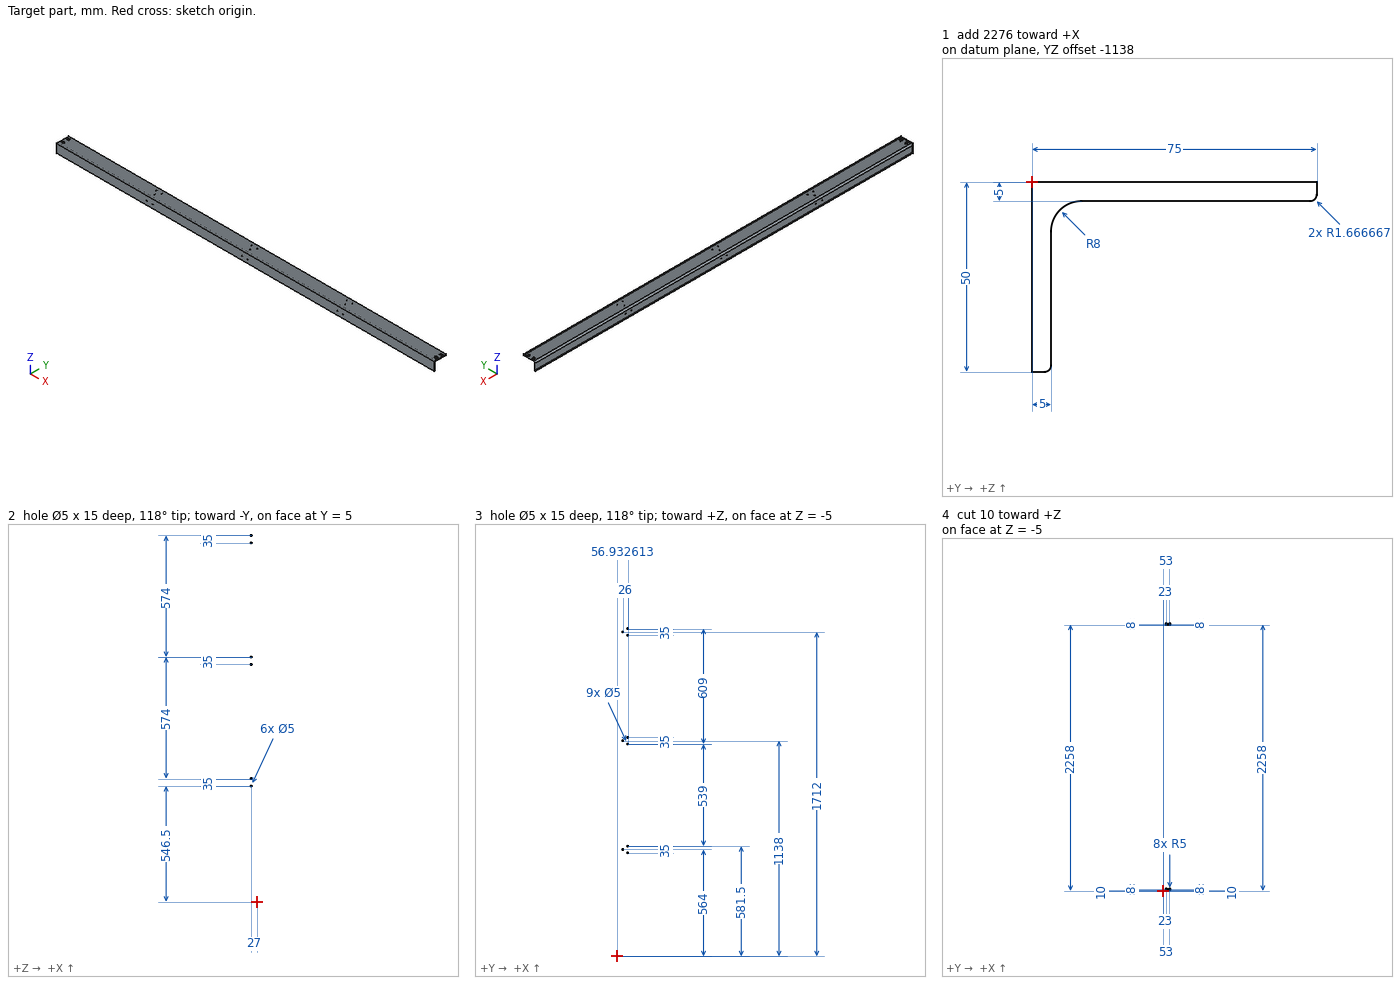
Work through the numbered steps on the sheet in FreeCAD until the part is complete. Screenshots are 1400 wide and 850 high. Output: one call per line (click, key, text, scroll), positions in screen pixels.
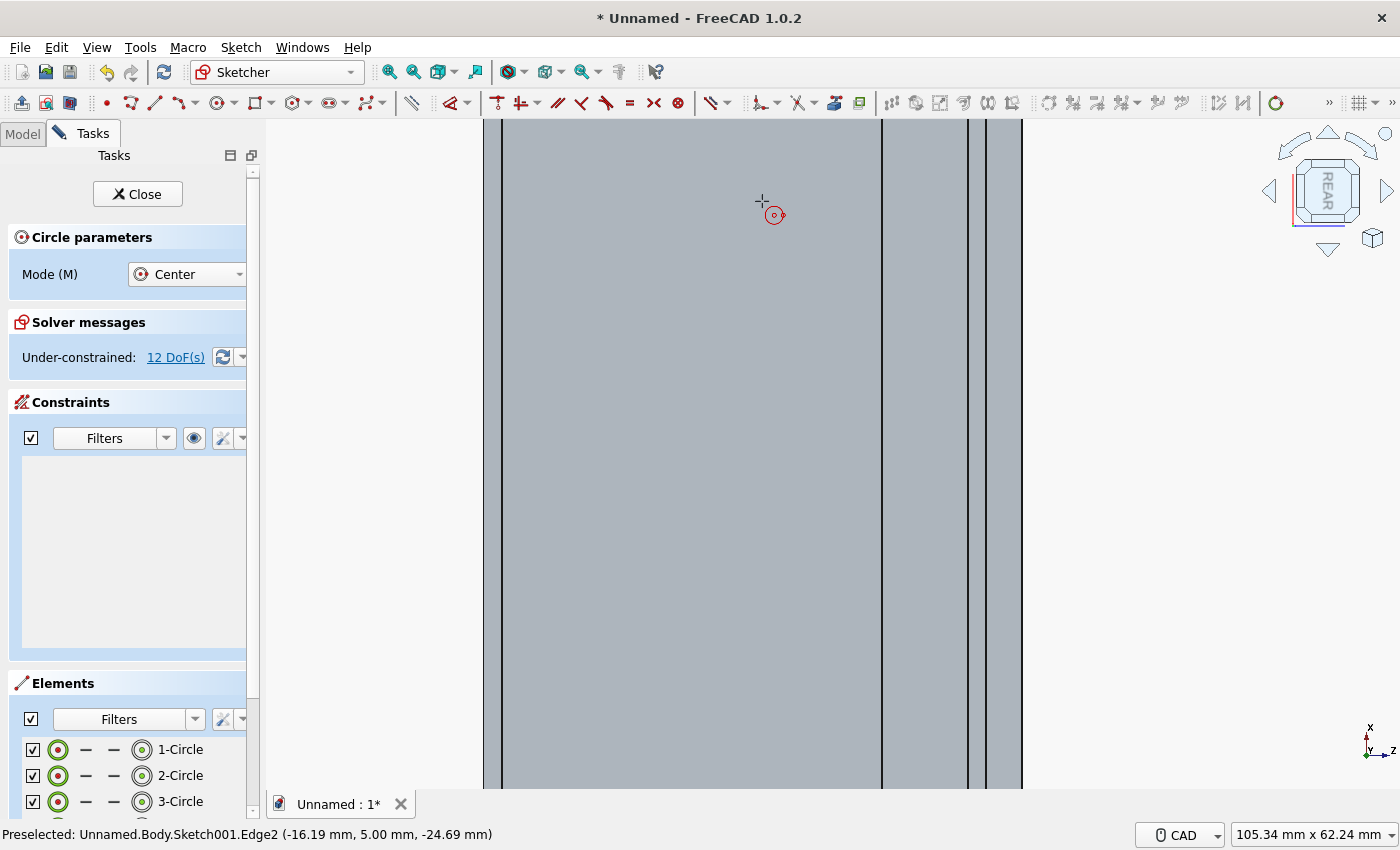
scroll(762, 200, down, 18)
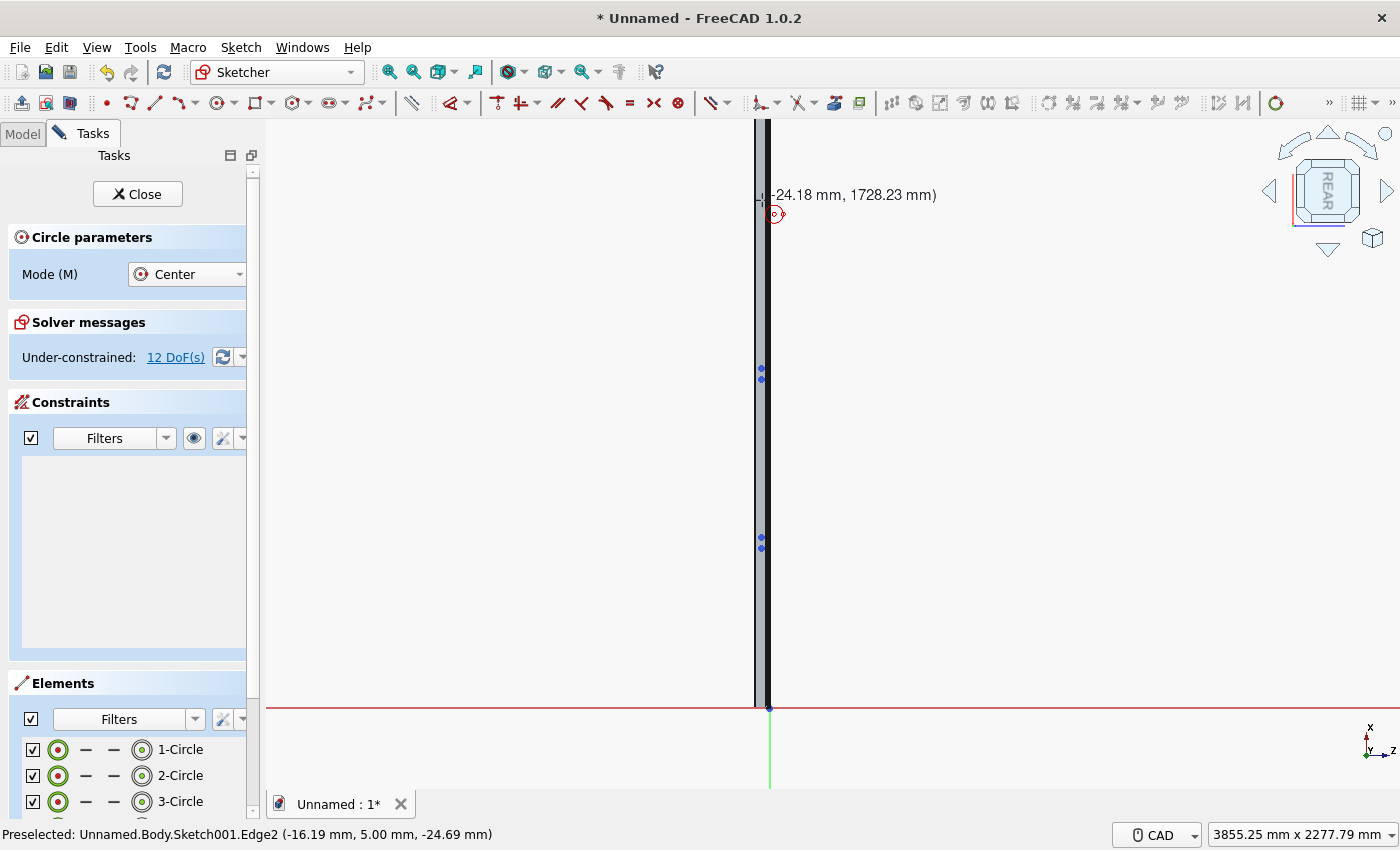
scroll(762, 200, up, 4)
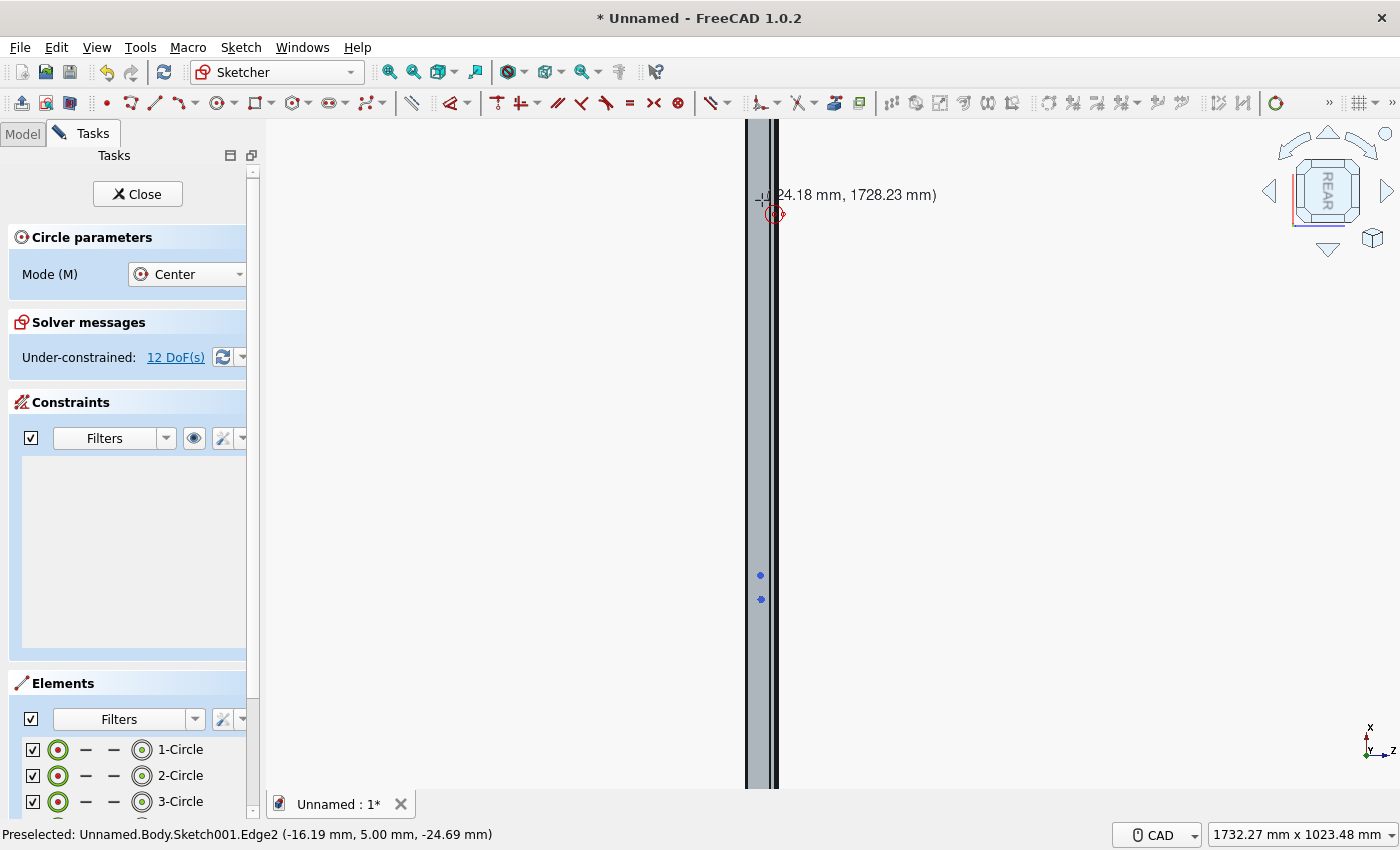
click(761, 199)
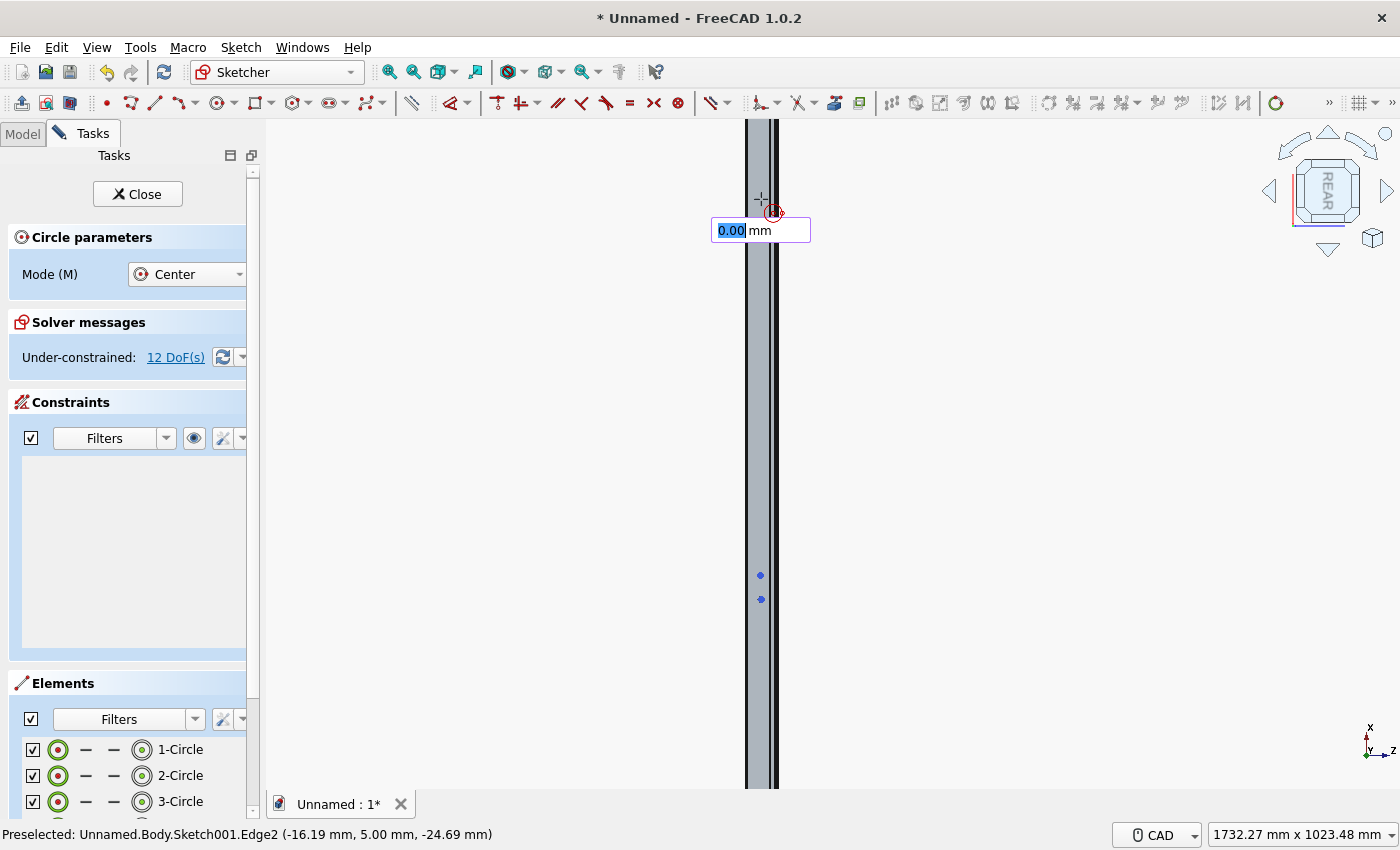
scroll(762, 198, up, 12)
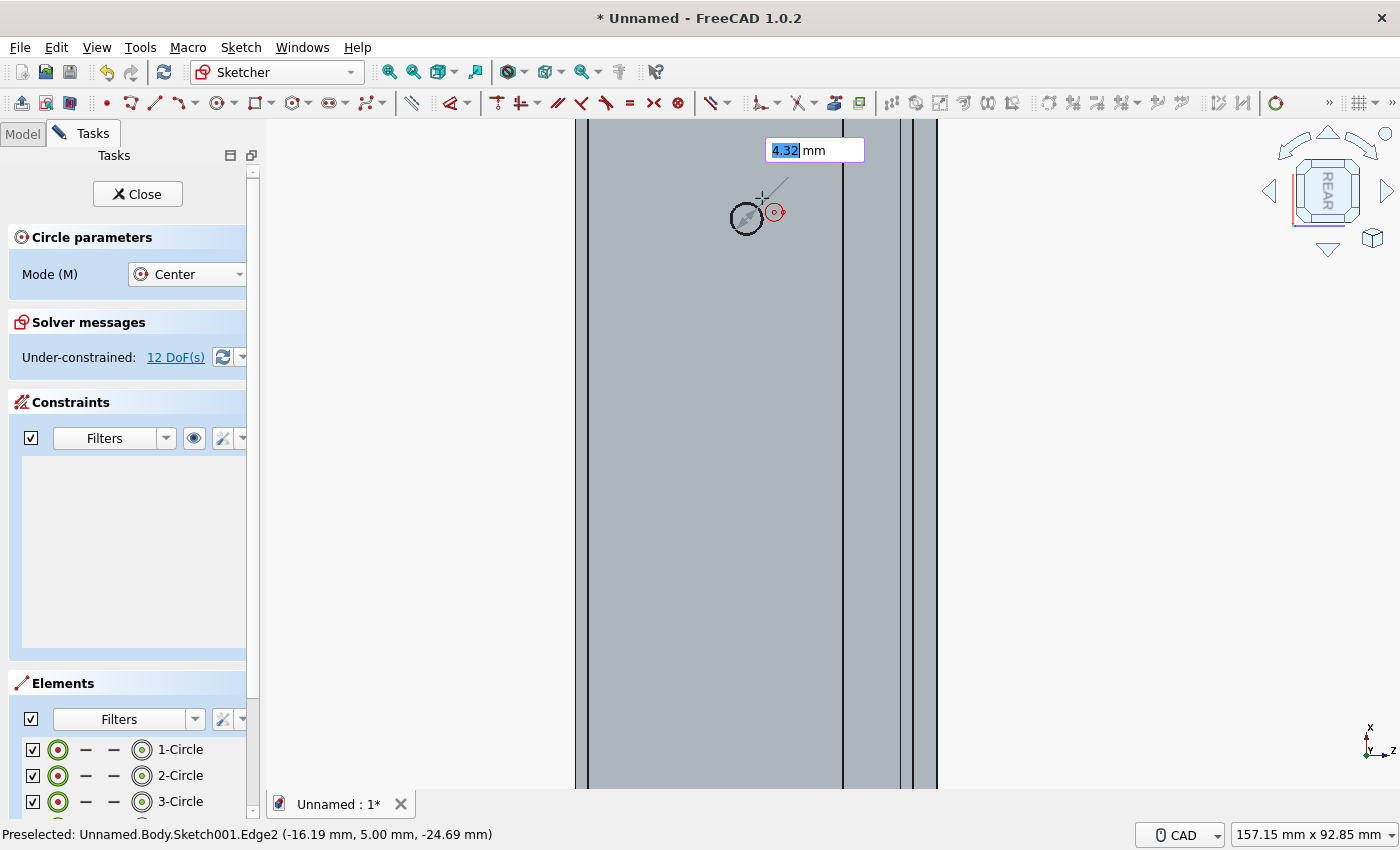
click(755, 199)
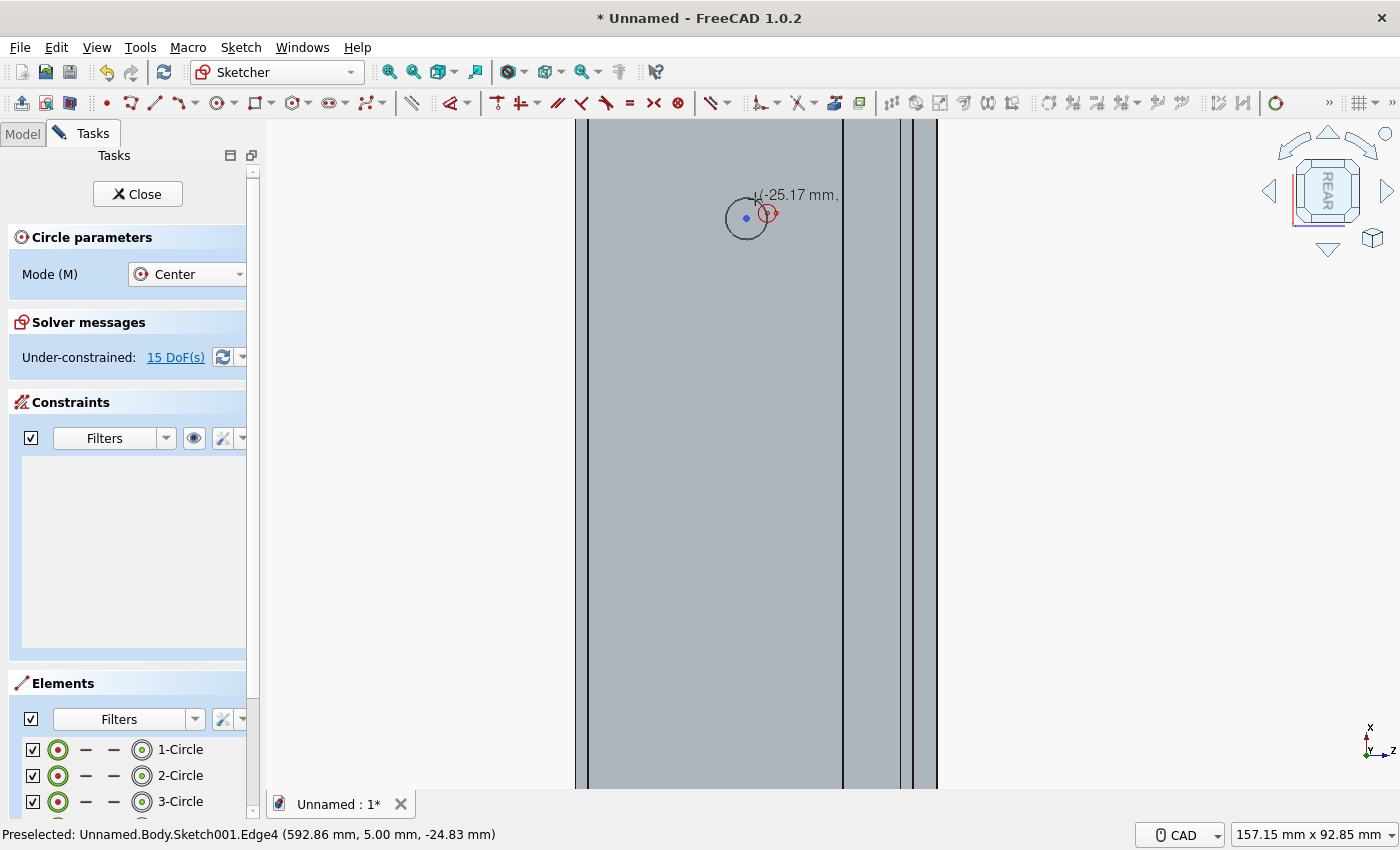
scroll(742, 464, up, 2)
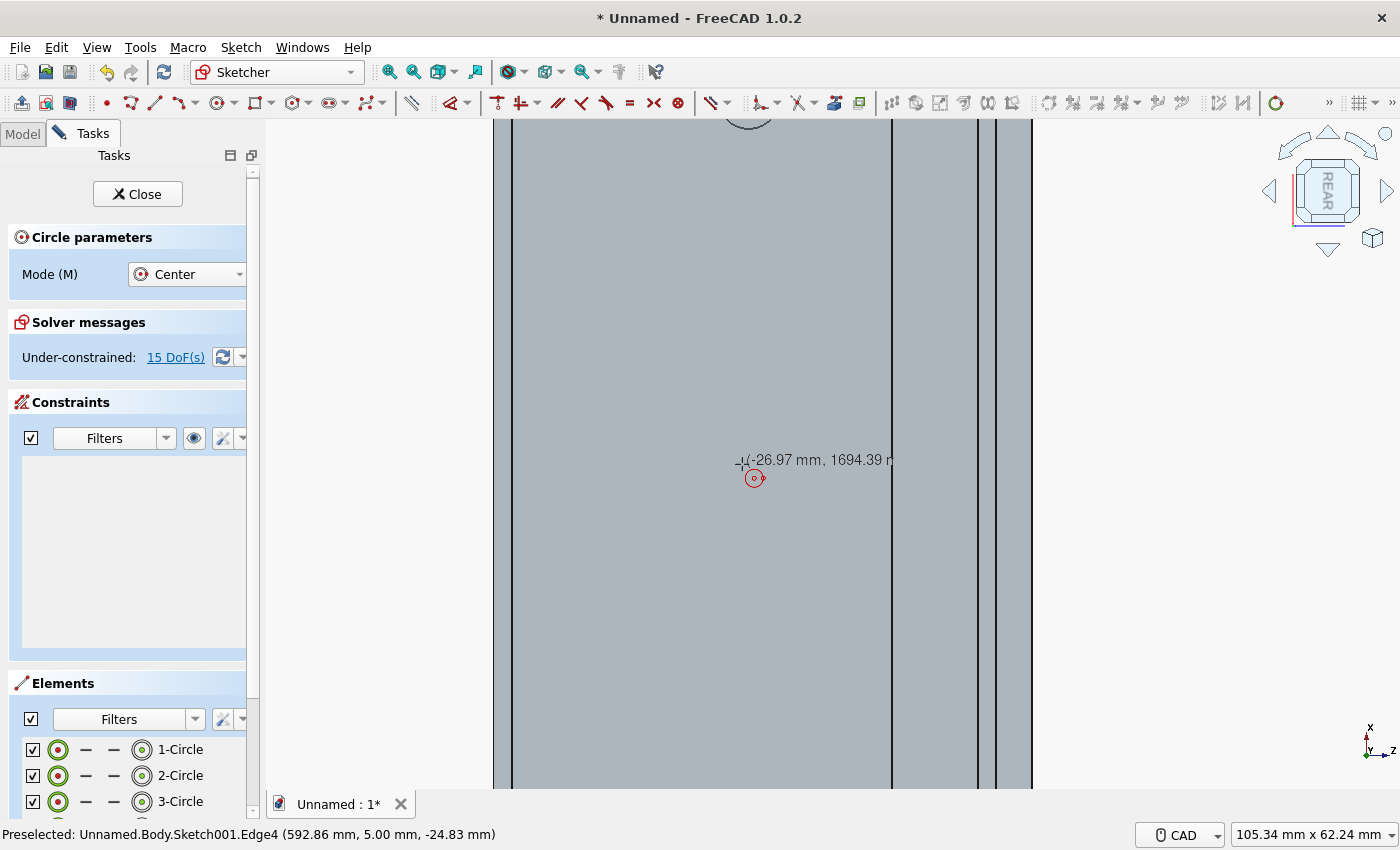
scroll(761, 203, down, 18)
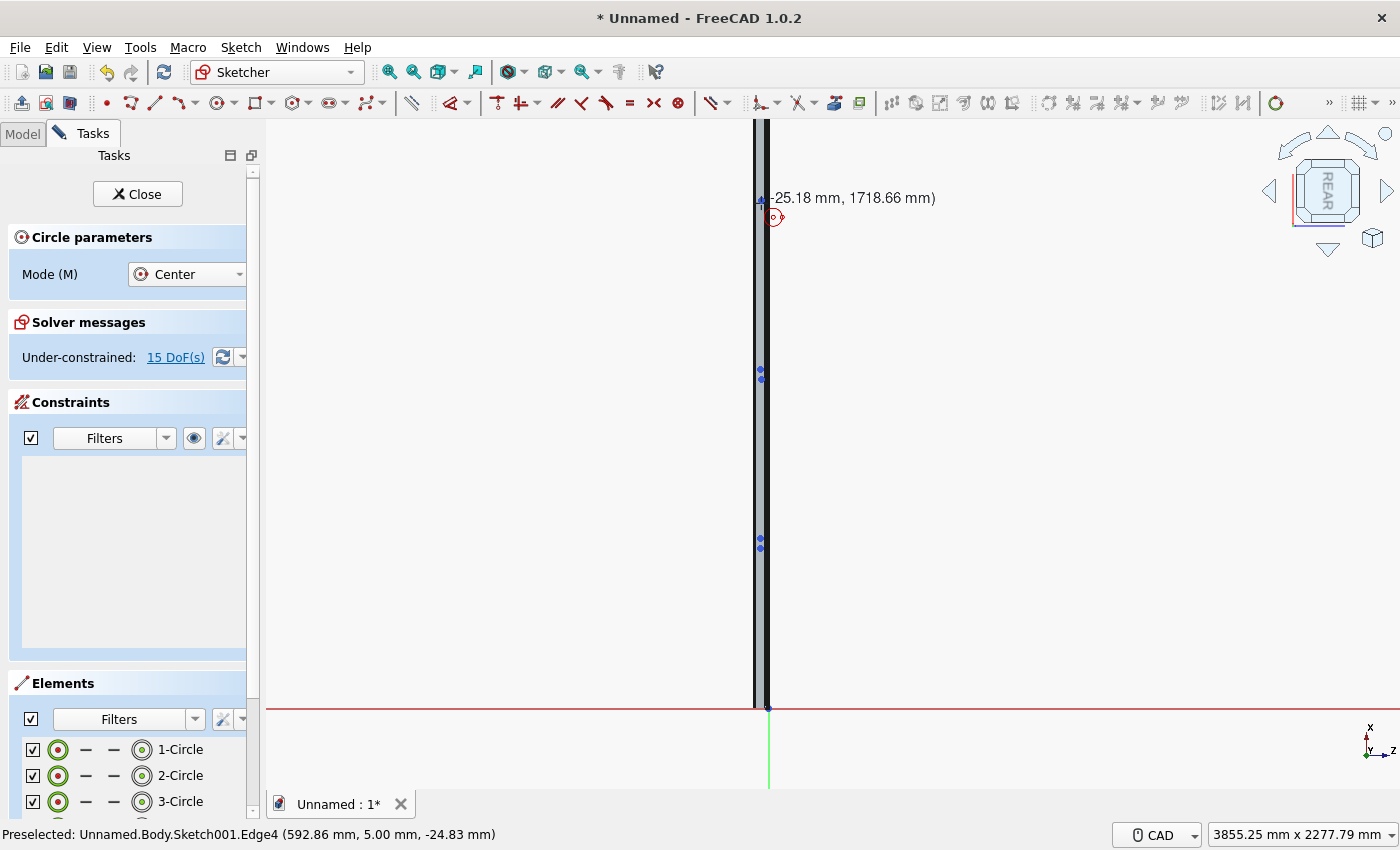
scroll(761, 210, up, 4)